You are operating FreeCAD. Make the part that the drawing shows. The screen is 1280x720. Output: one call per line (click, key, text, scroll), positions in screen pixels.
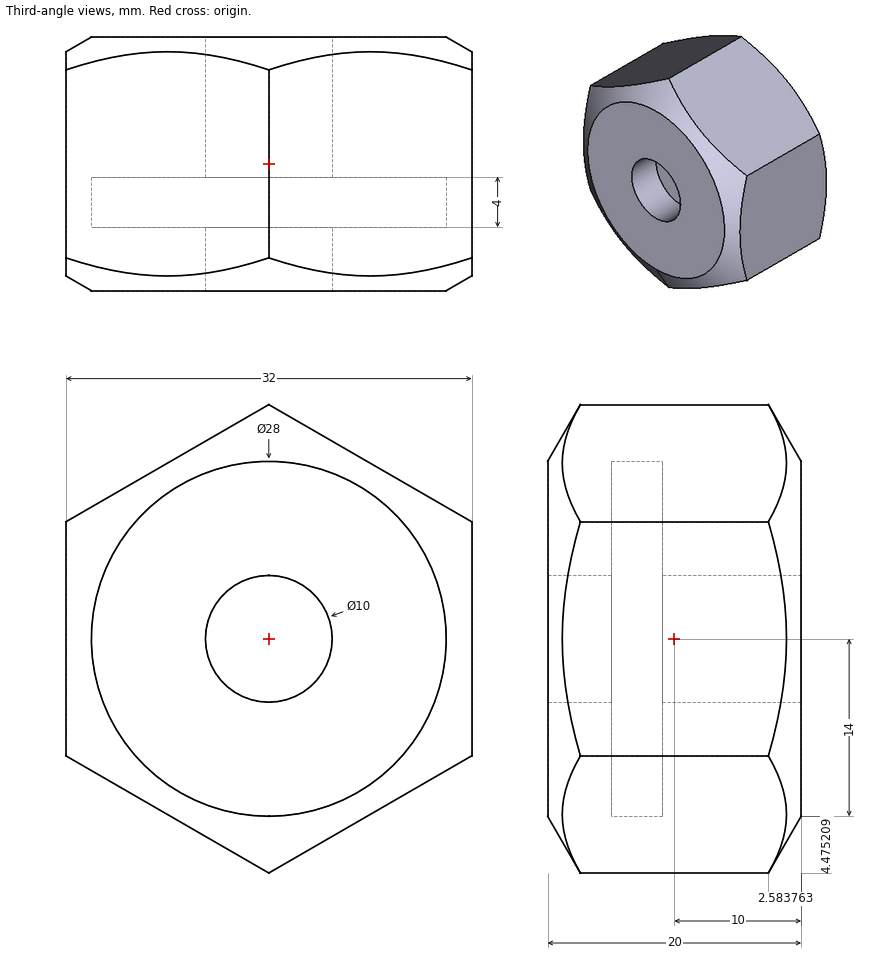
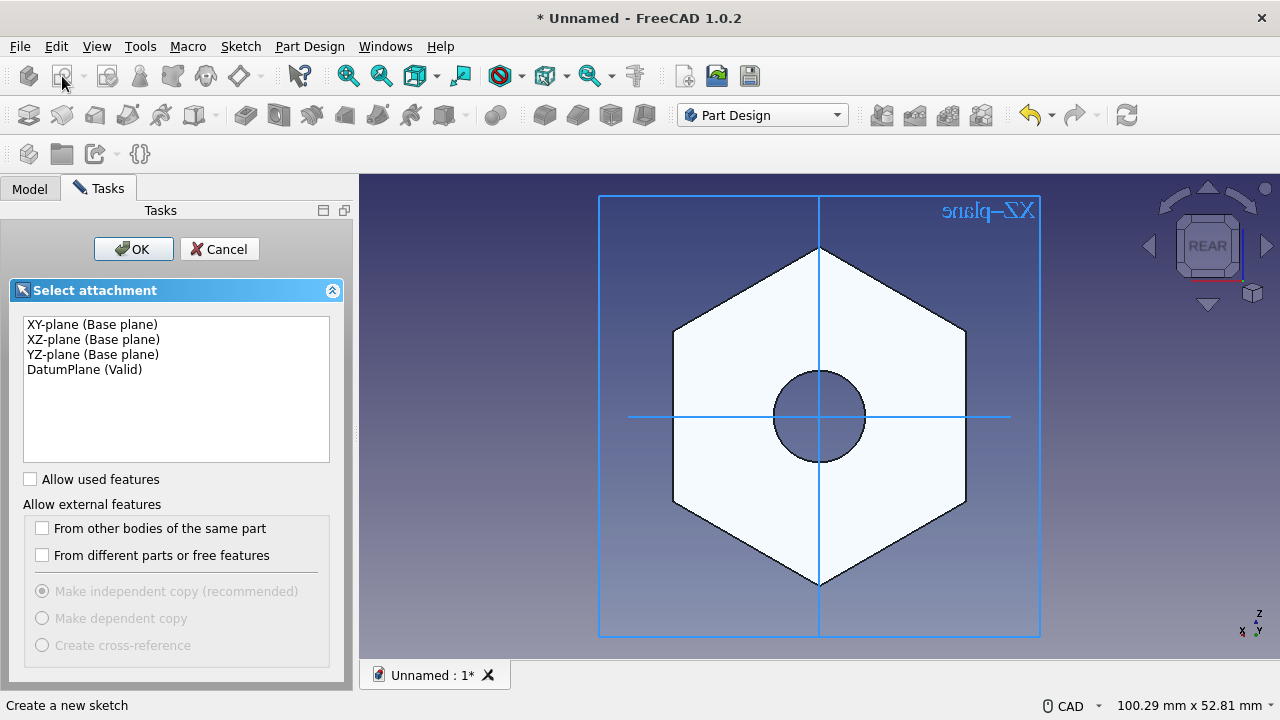
click(84, 354)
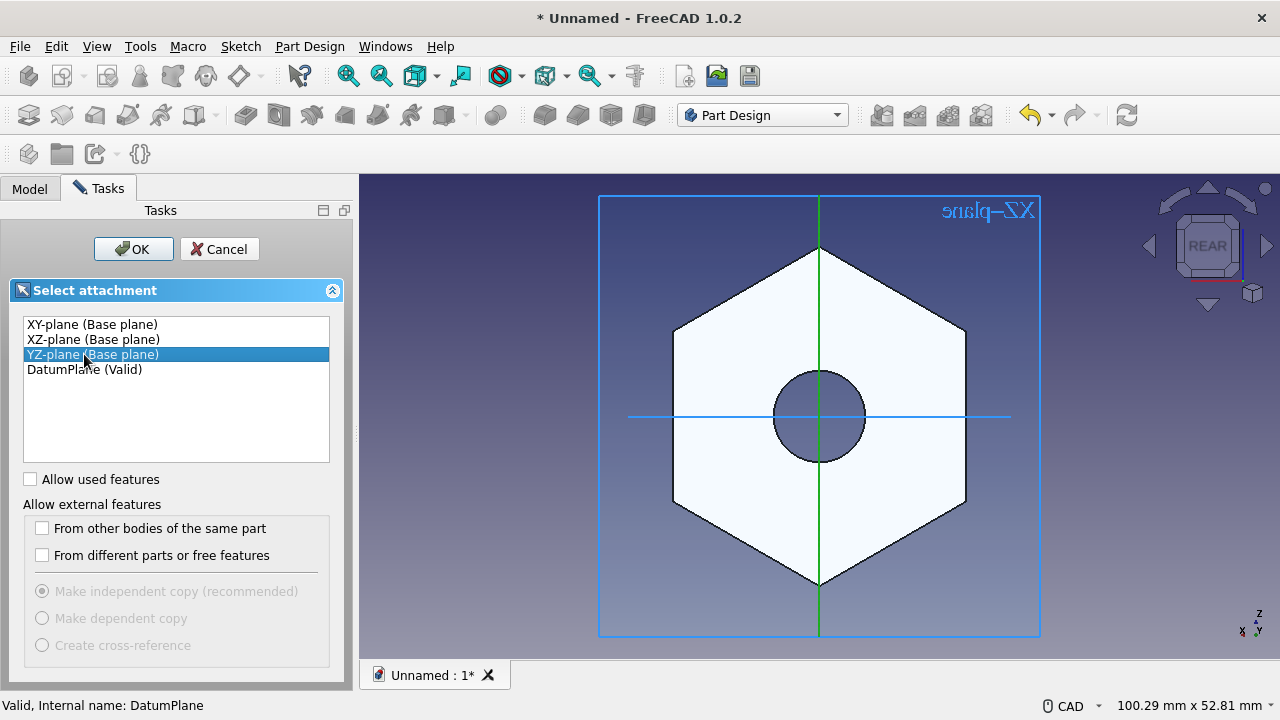
click(134, 249)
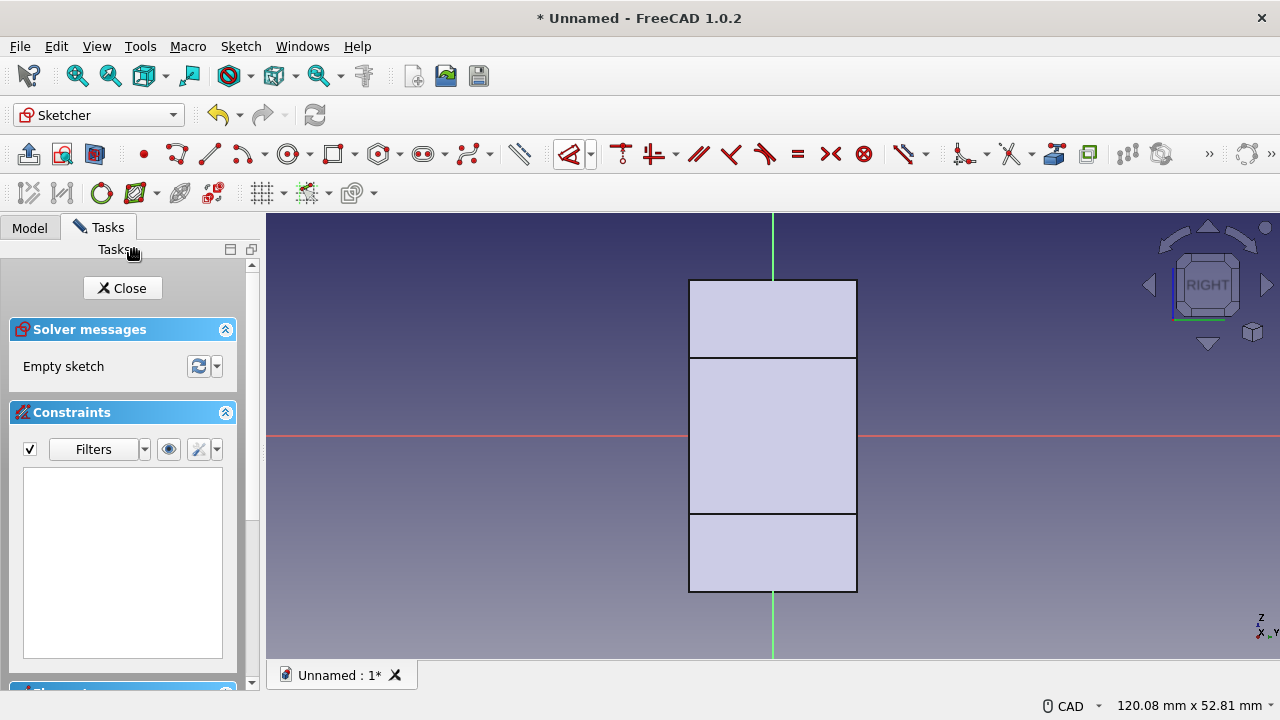
click(95, 154)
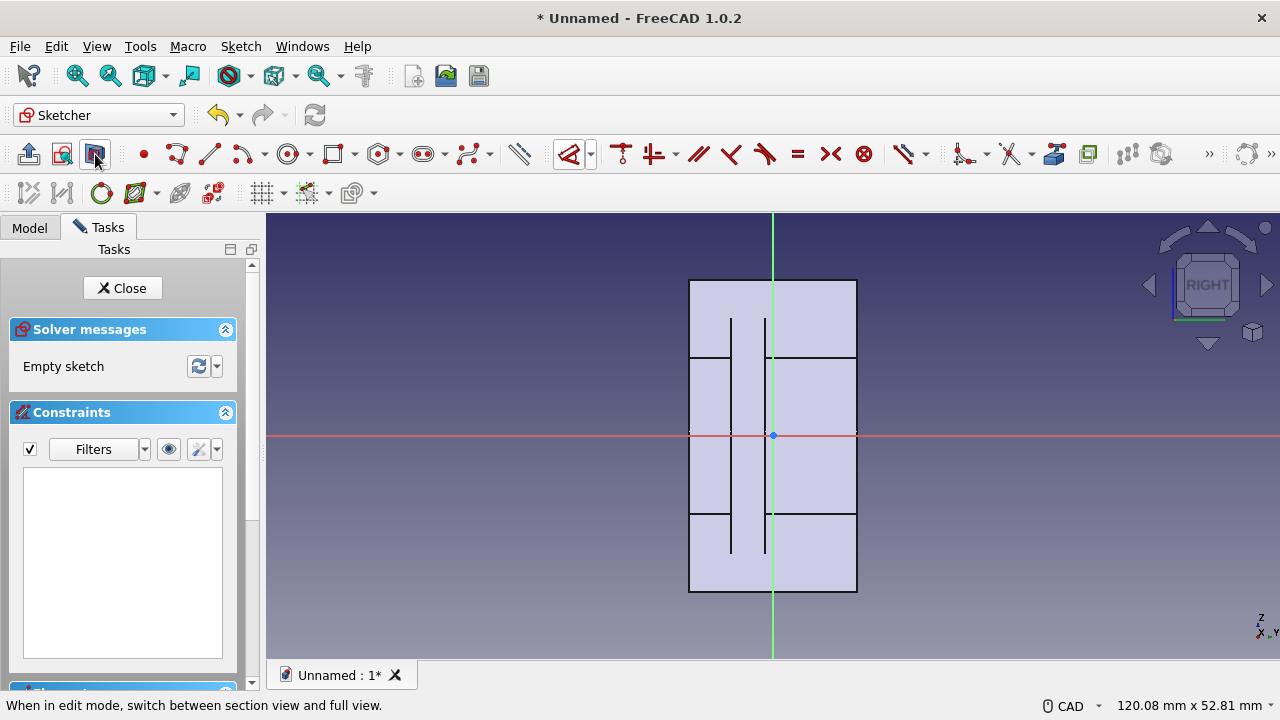
scroll(869, 595, up, 10)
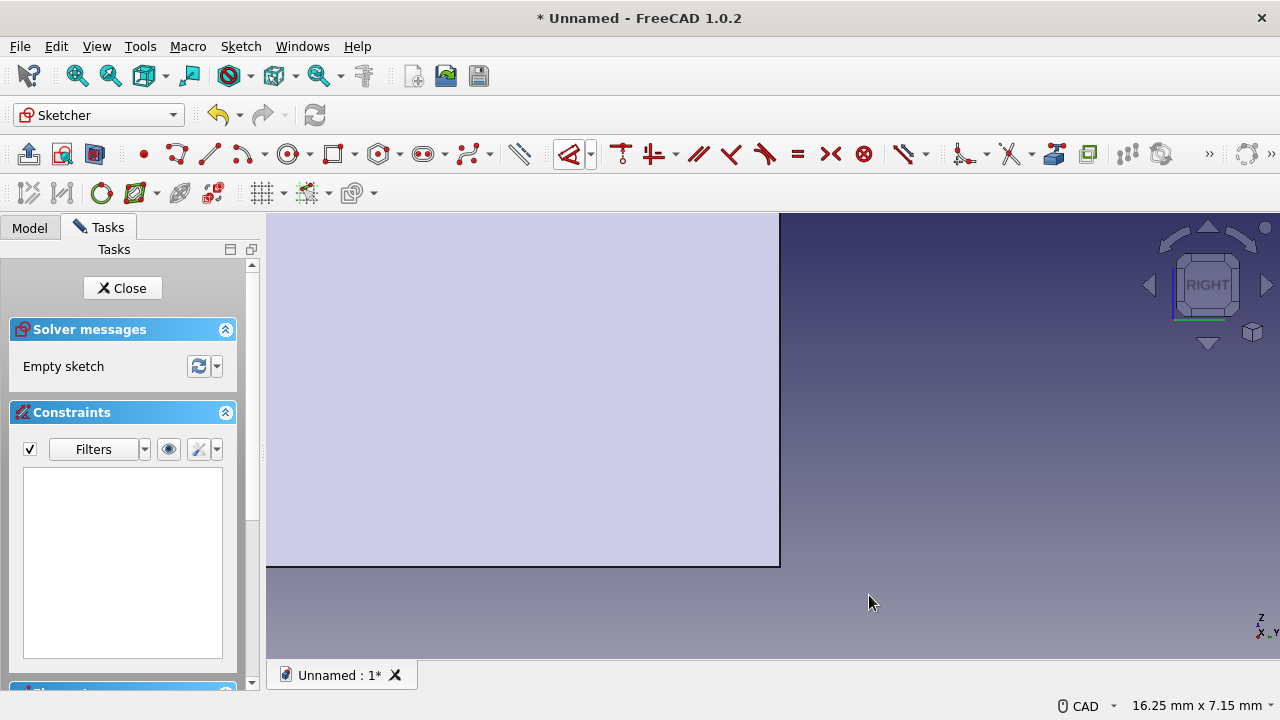
click(177, 154)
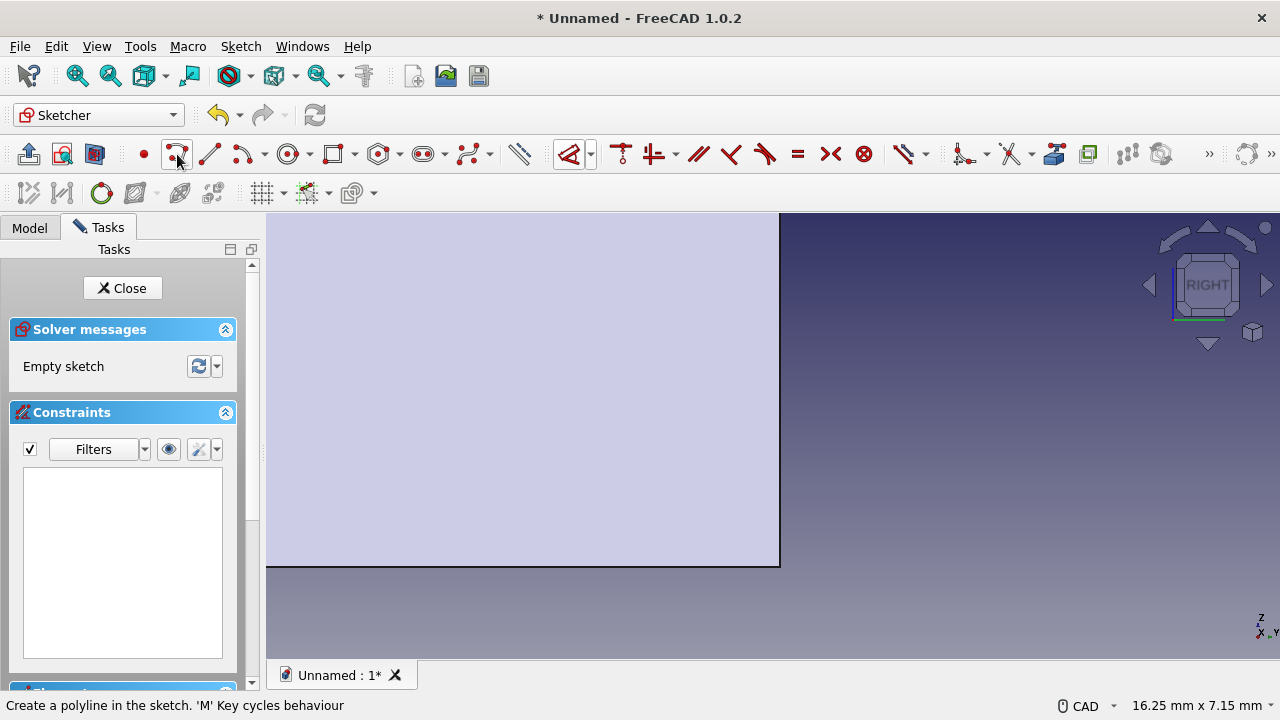
click(780, 288)
click(619, 567)
click(780, 567)
click(780, 289)
key(Escape)
key(Escape)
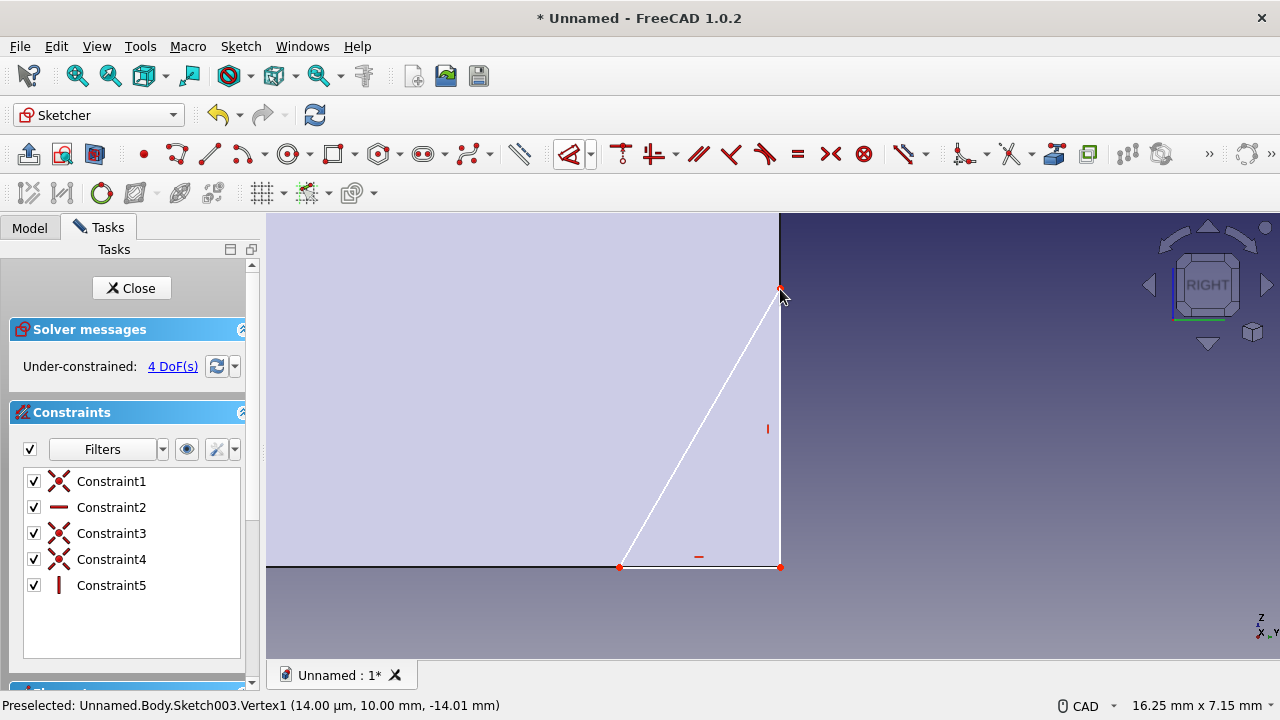
click(780, 289)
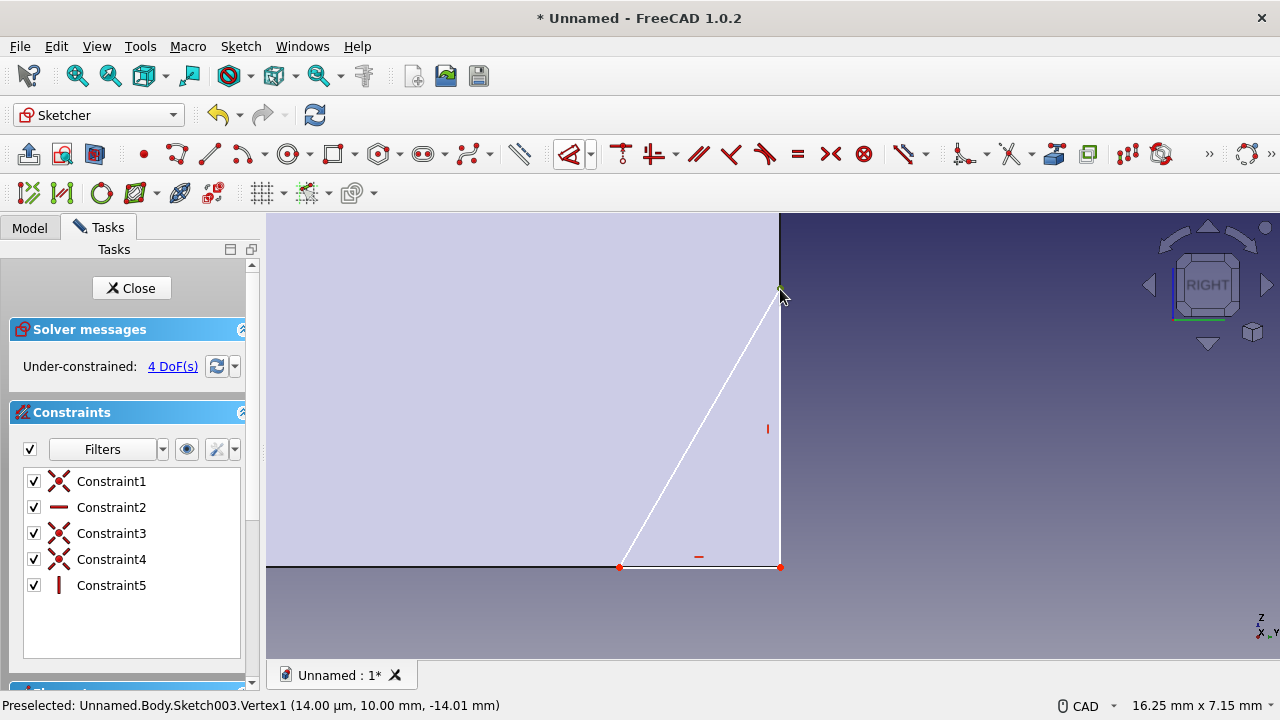
click(590, 154)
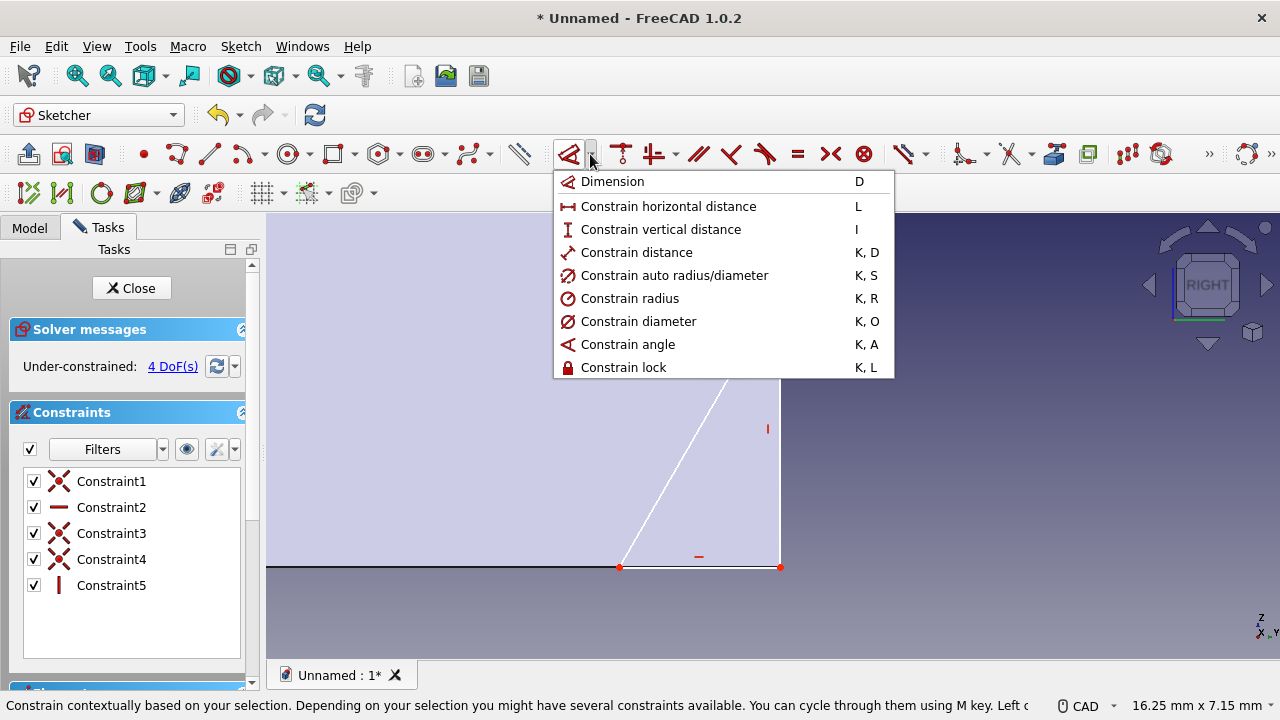
click(724, 206)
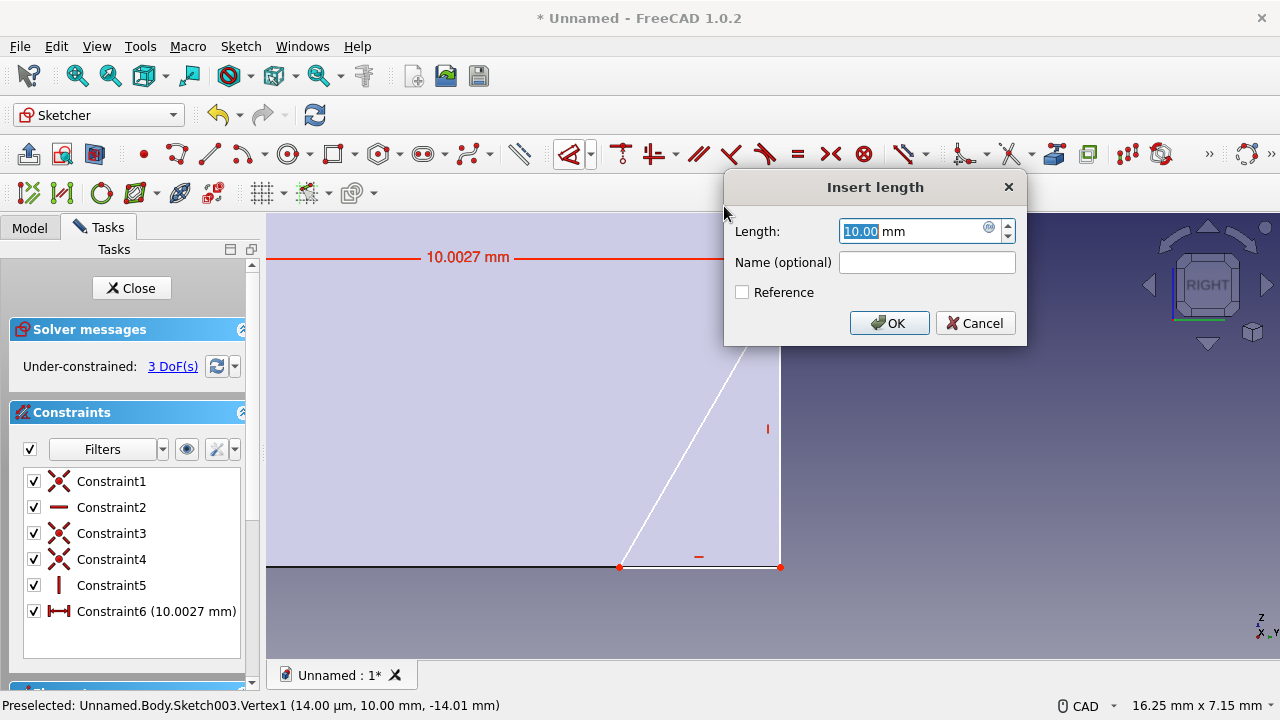
text(10)
key(Return)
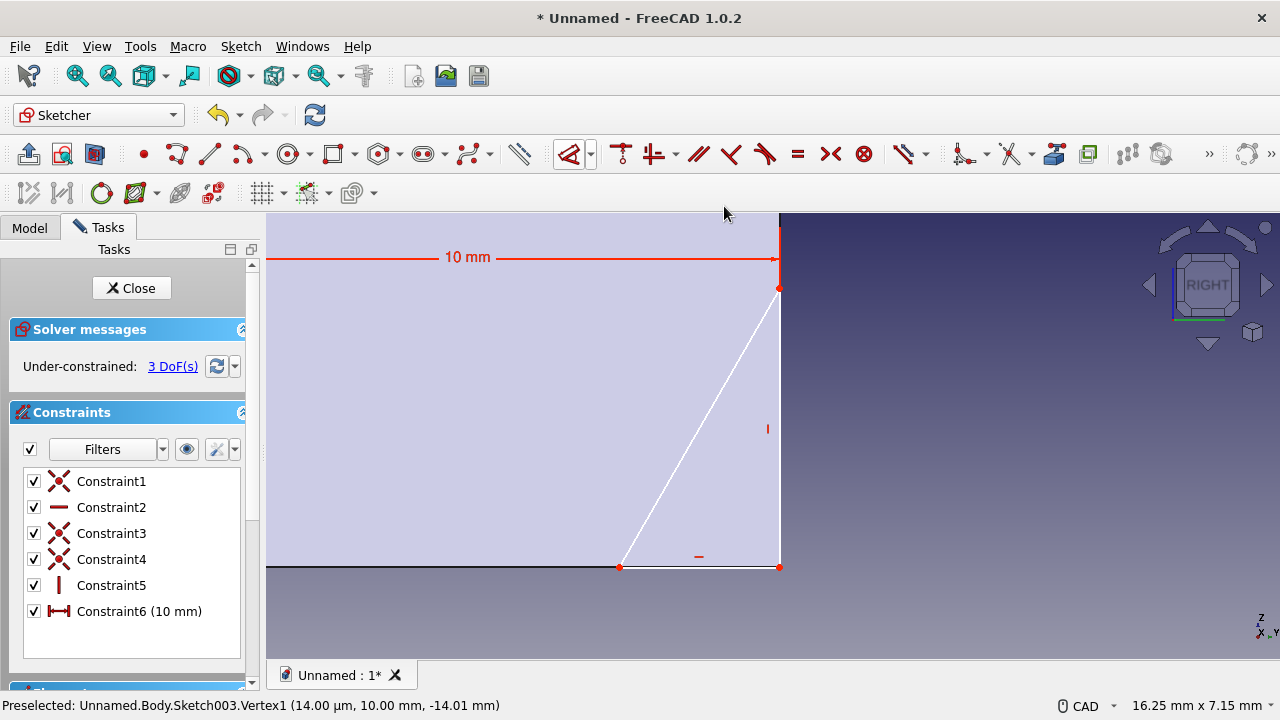
click(780, 289)